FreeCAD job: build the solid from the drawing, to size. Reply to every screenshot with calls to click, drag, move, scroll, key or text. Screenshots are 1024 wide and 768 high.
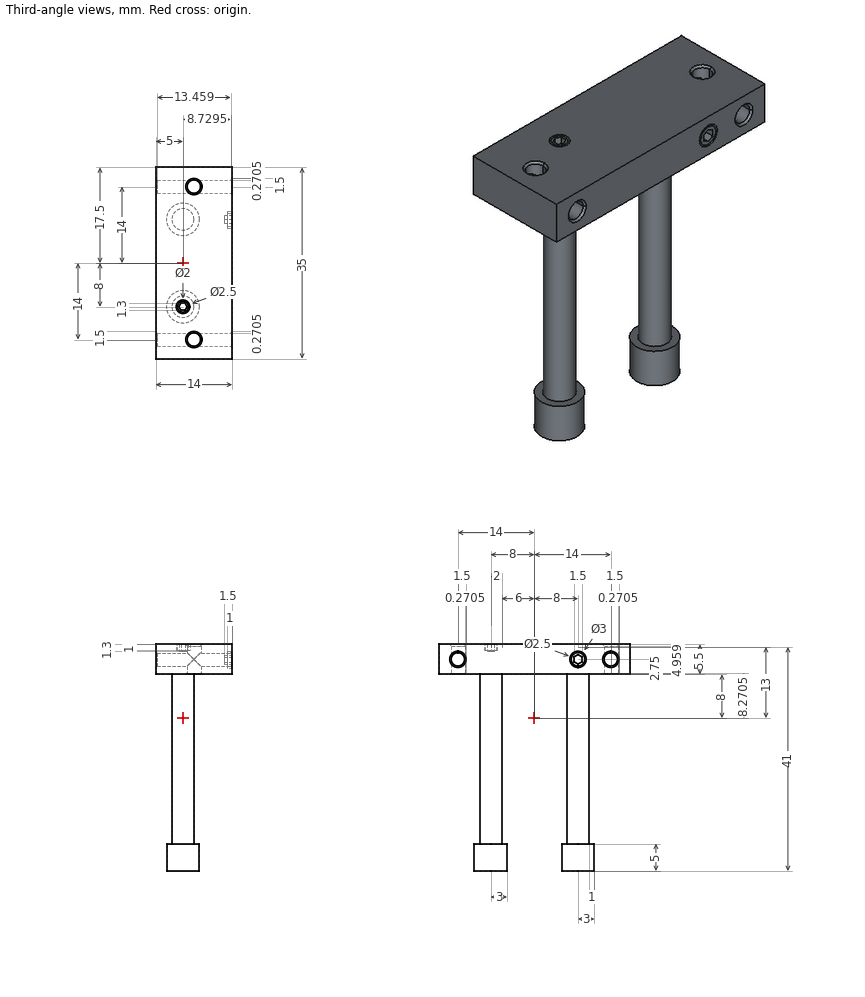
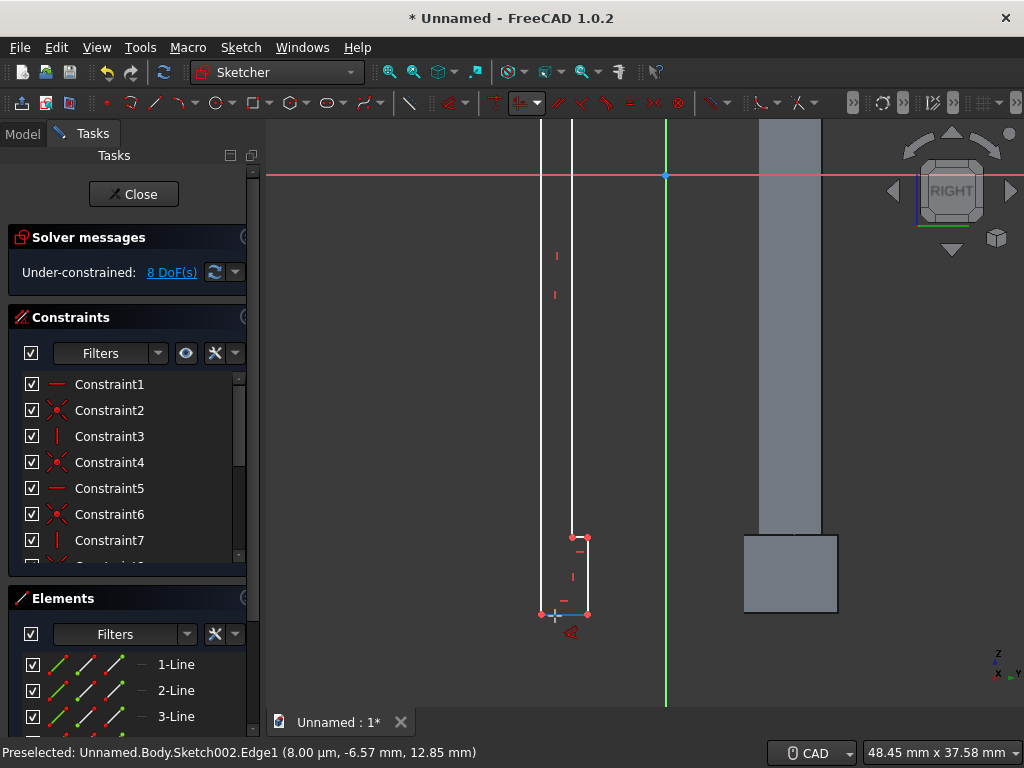
click(555, 615)
click(565, 649)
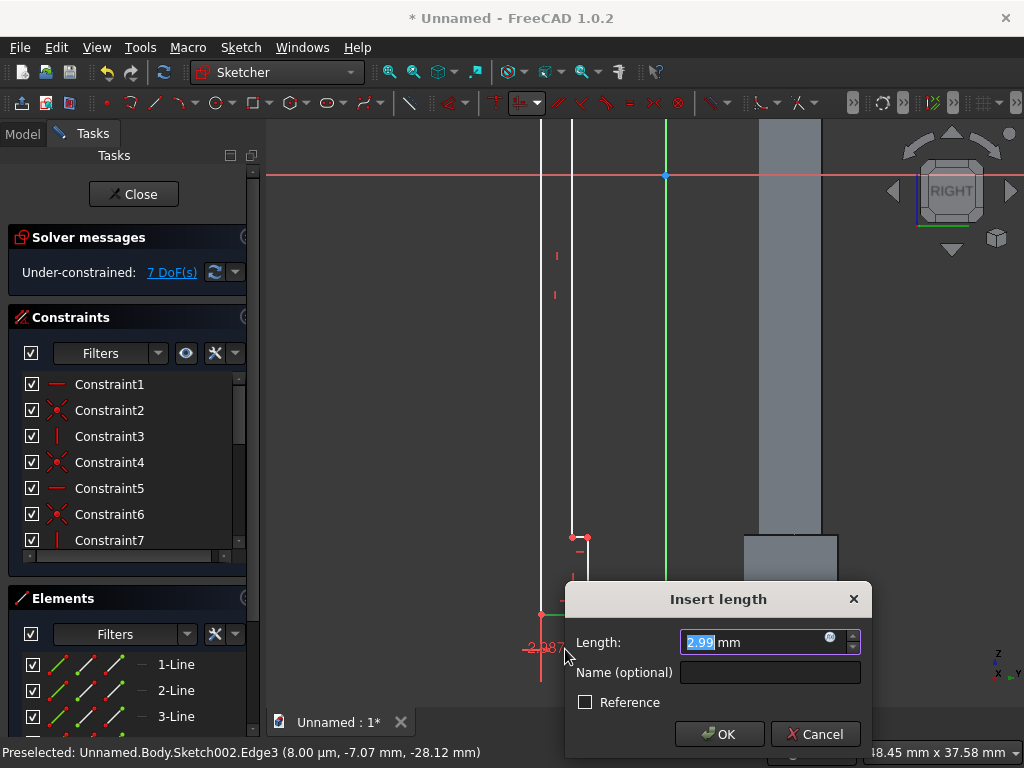
text(3)
key(Return)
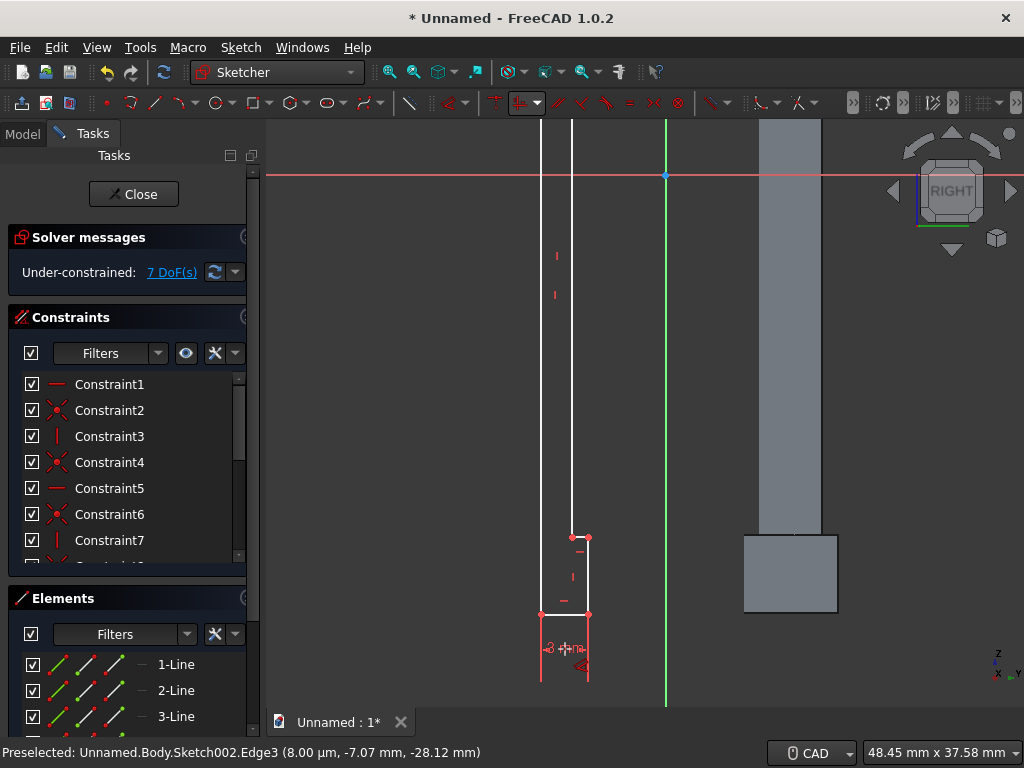
click(588, 592)
click(622, 576)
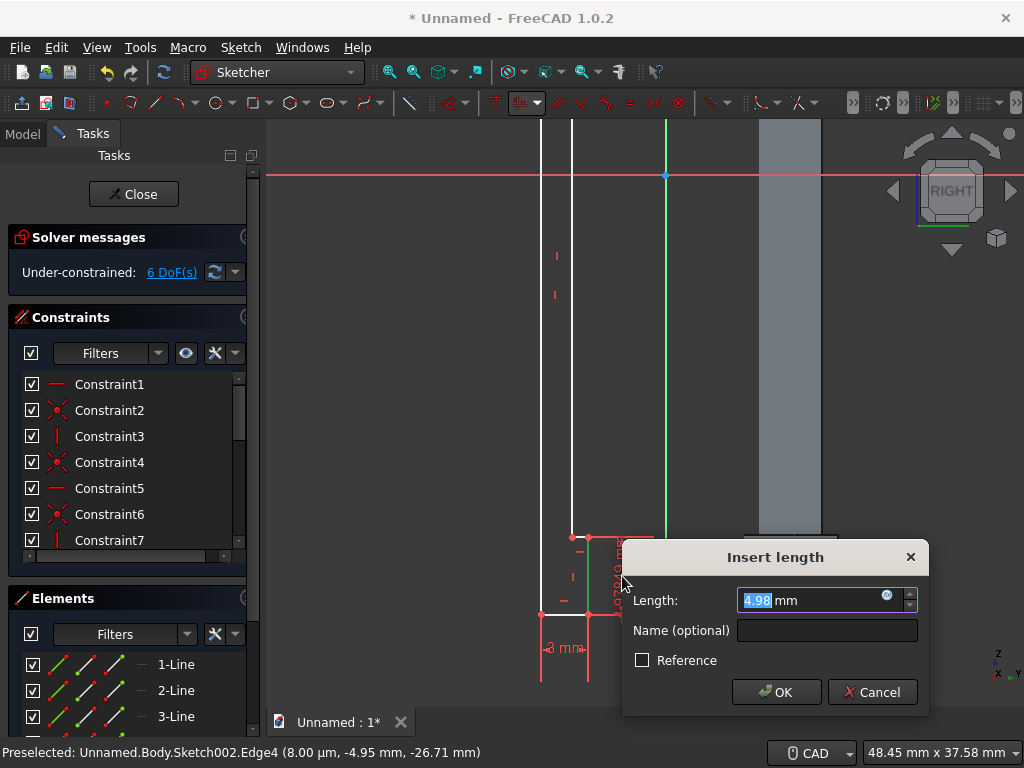
text(5)
key(Return)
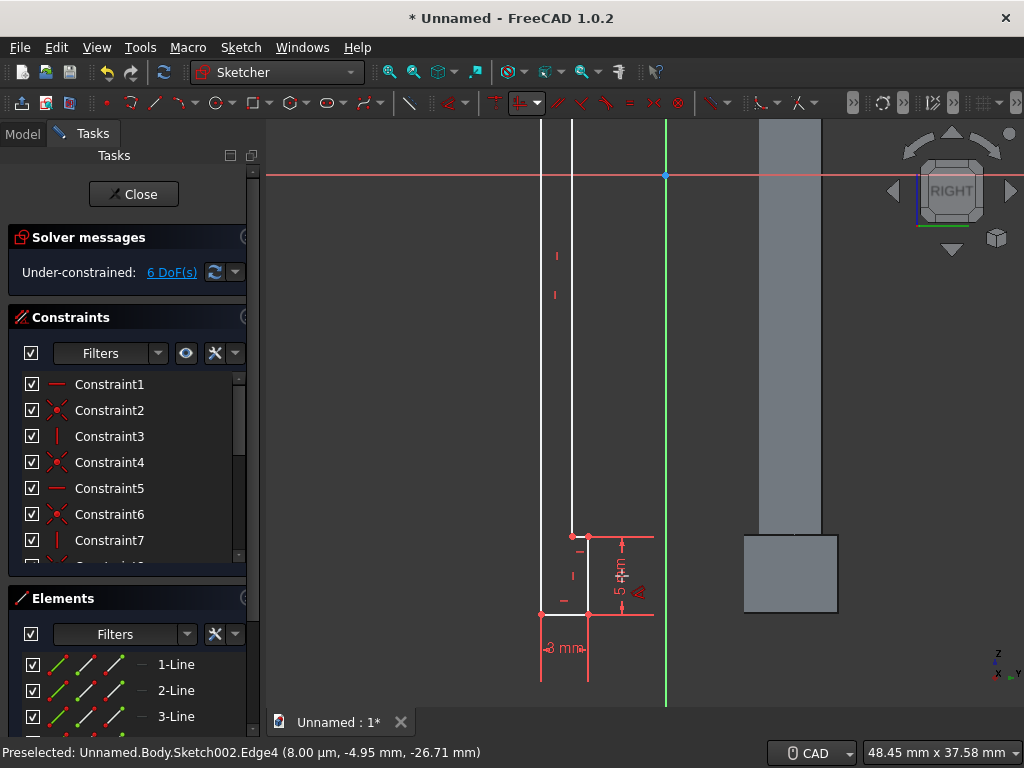
click(541, 423)
click(507, 381)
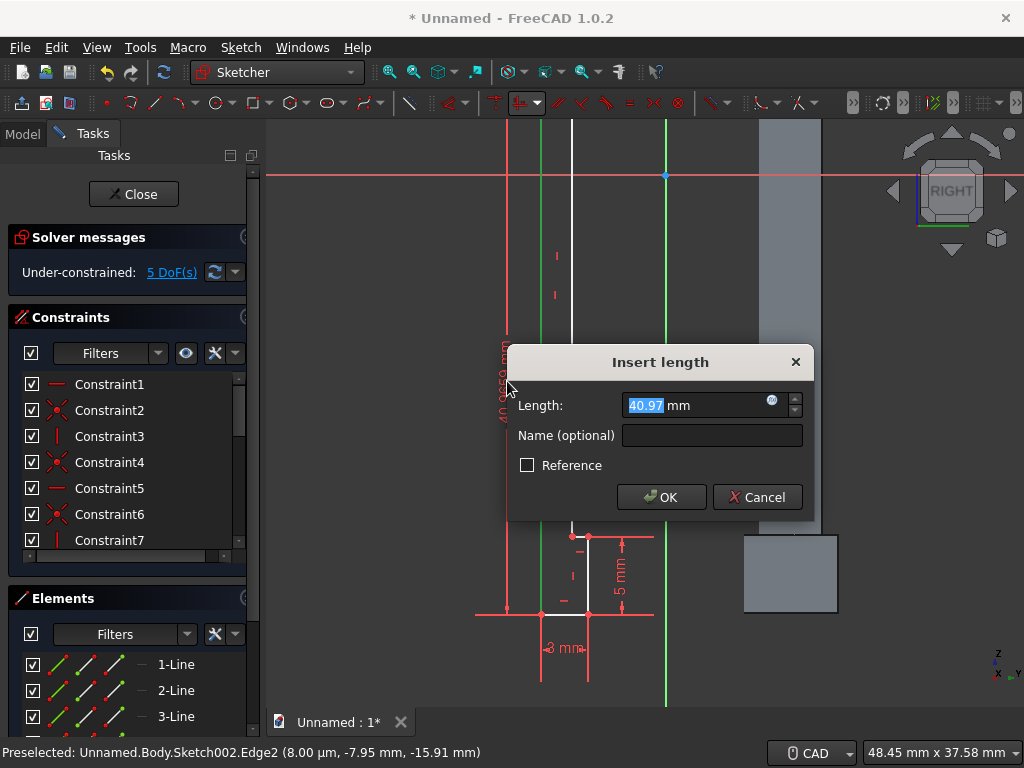
text(41)
key(Return)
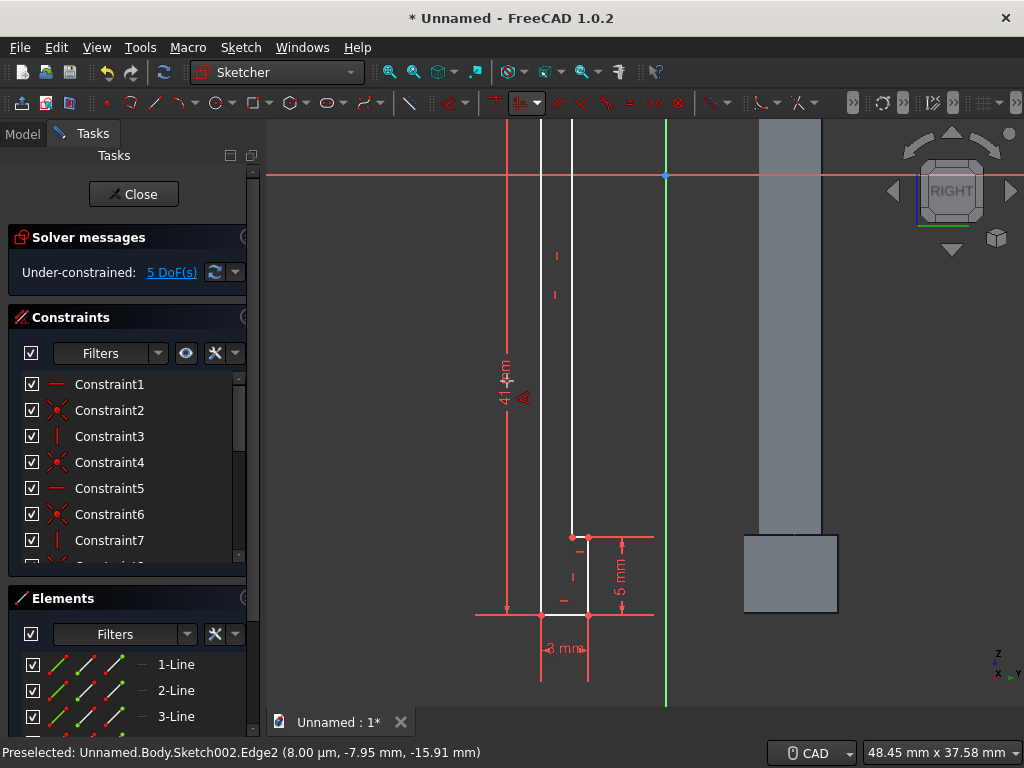
scroll(555, 616, down, 4)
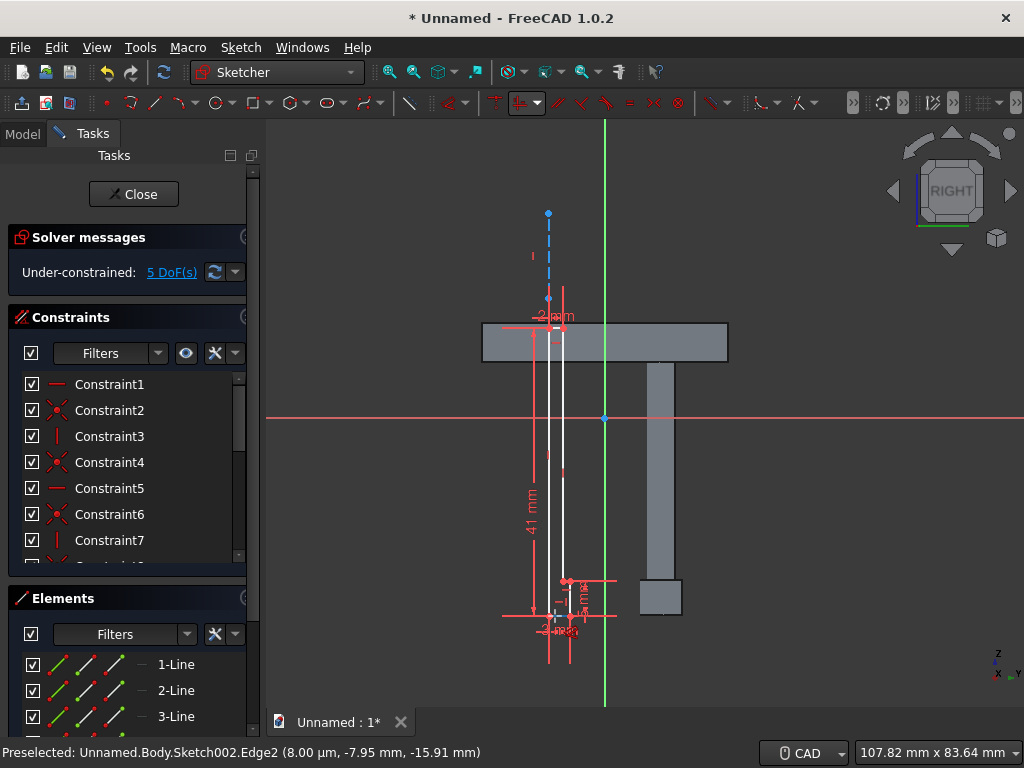
click(563, 328)
click(584, 294)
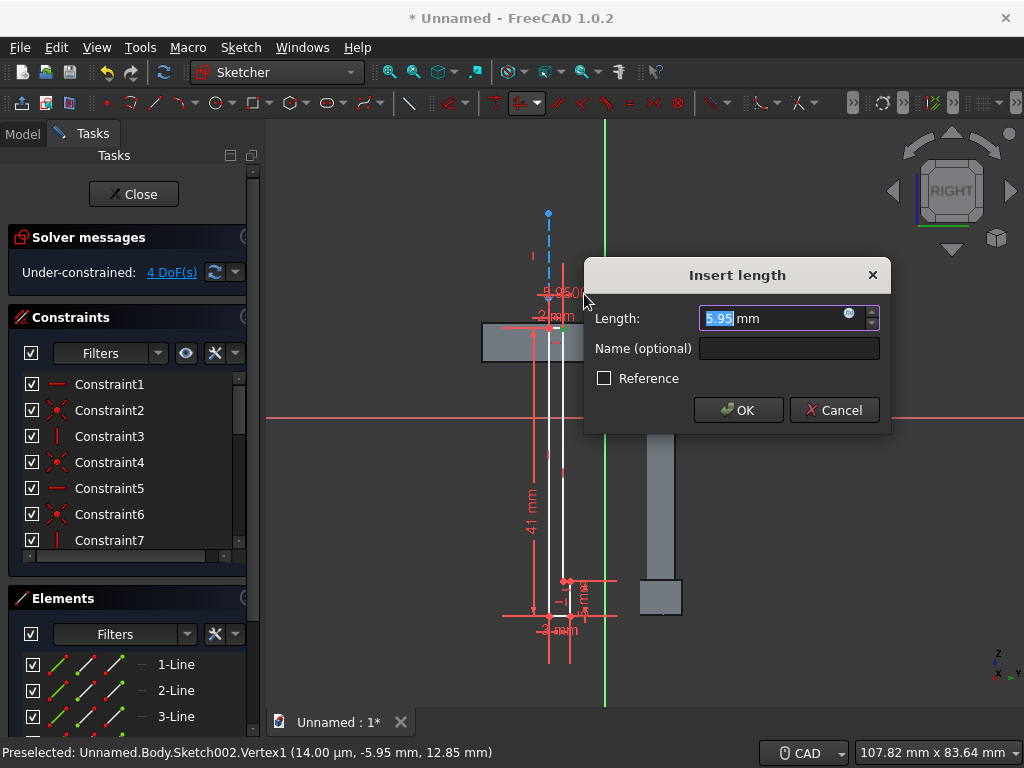
text(6)
key(Return)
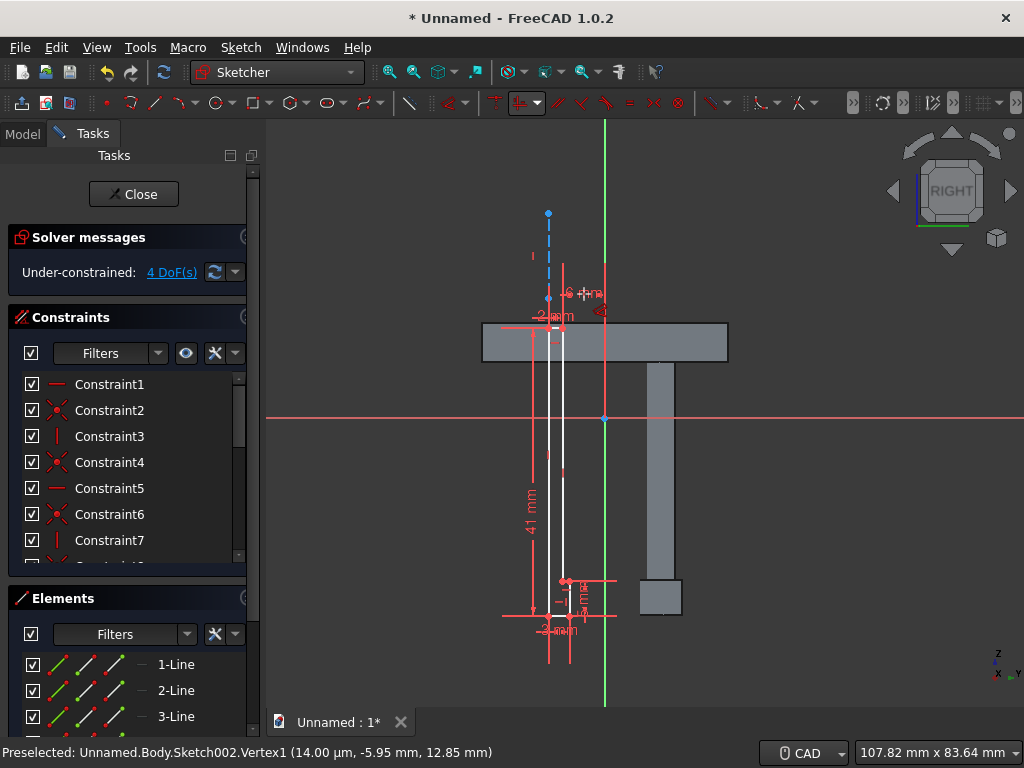
click(549, 299)
click(577, 265)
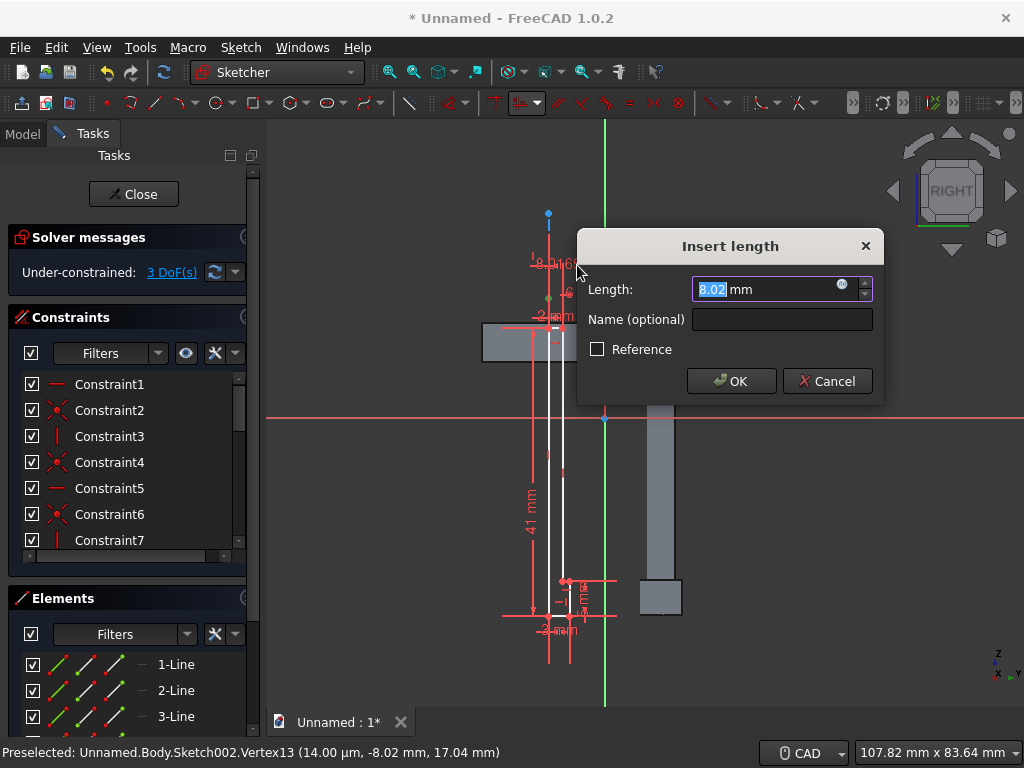
text(8)
key(Return)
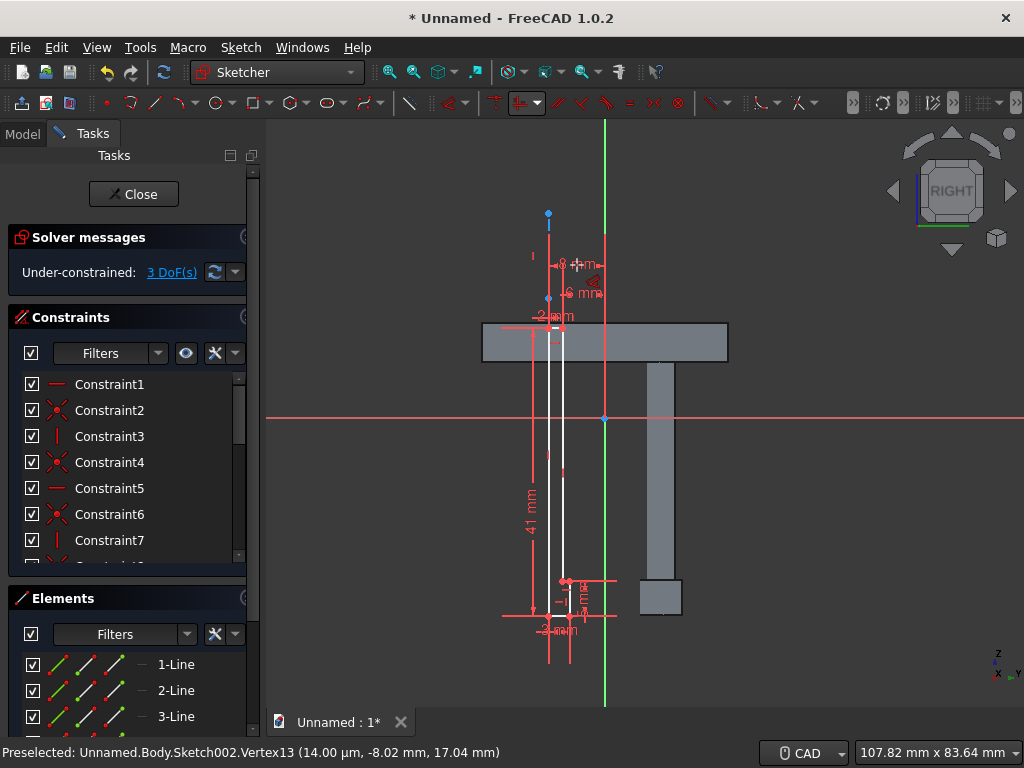
click(563, 328)
click(639, 373)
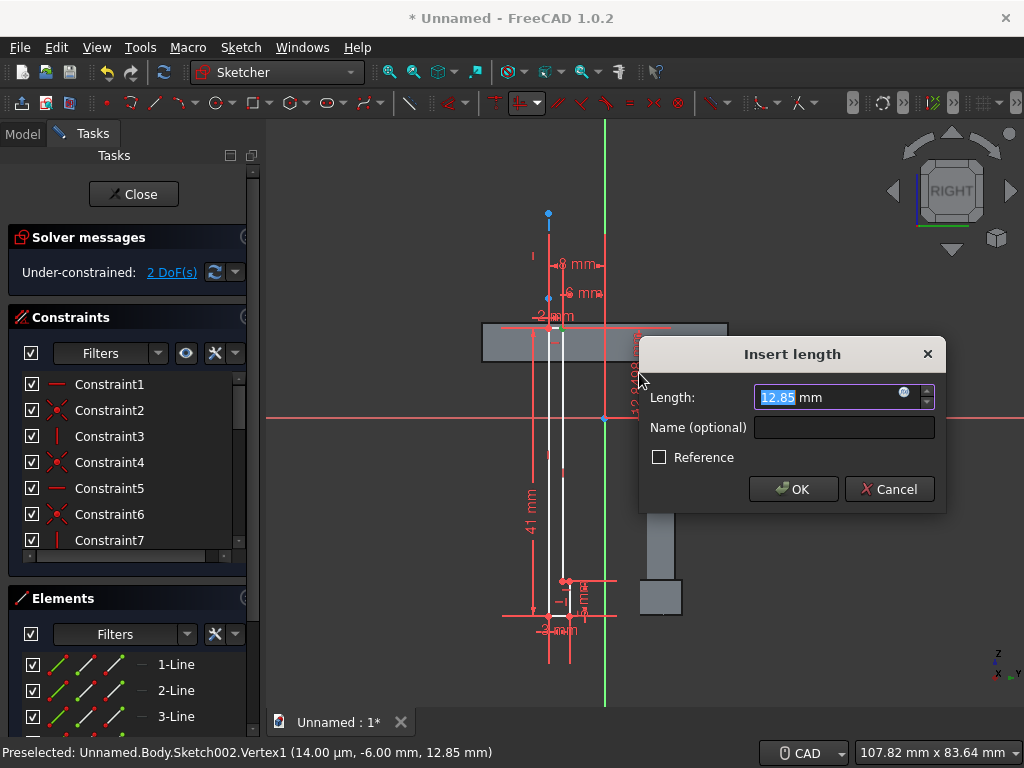
text(13)
key(Return)
key(Escape)